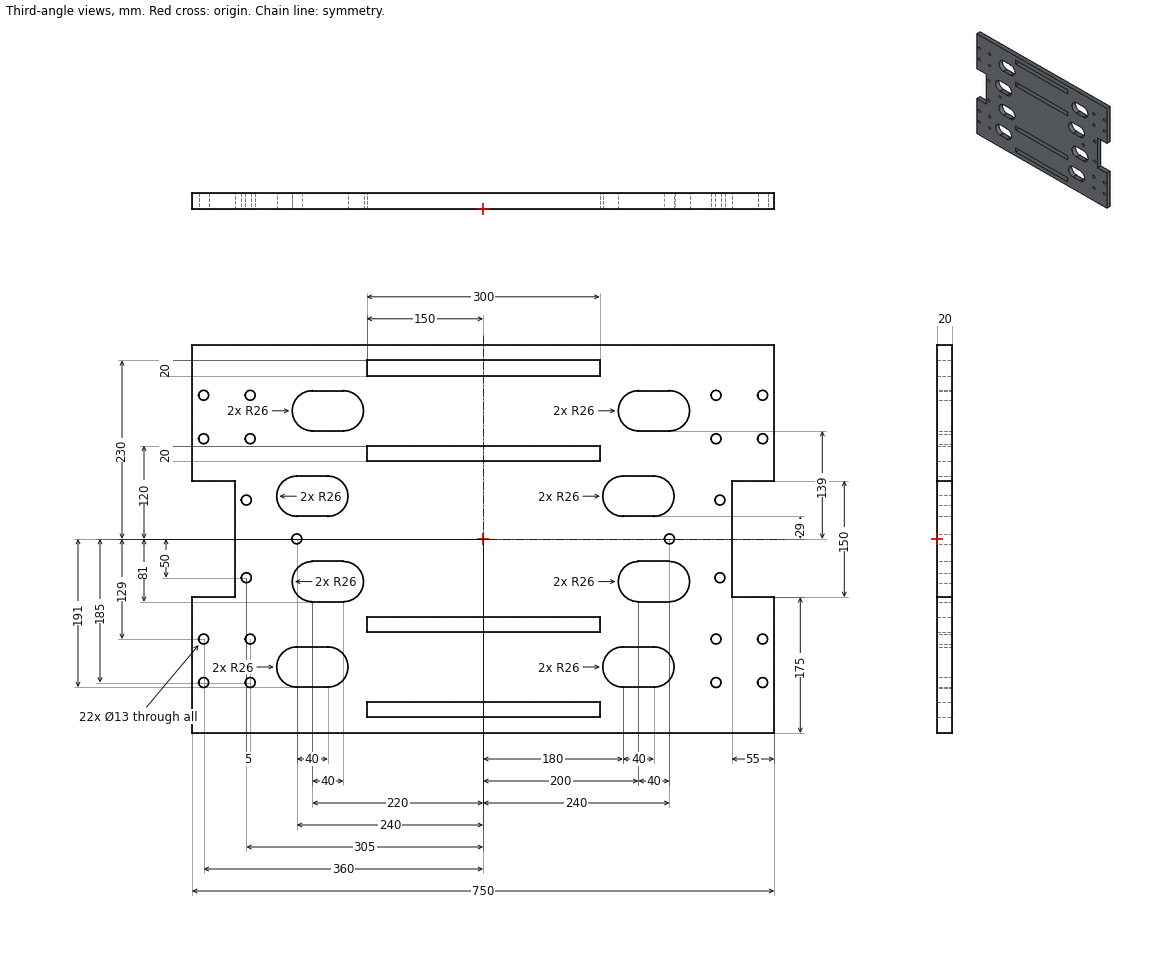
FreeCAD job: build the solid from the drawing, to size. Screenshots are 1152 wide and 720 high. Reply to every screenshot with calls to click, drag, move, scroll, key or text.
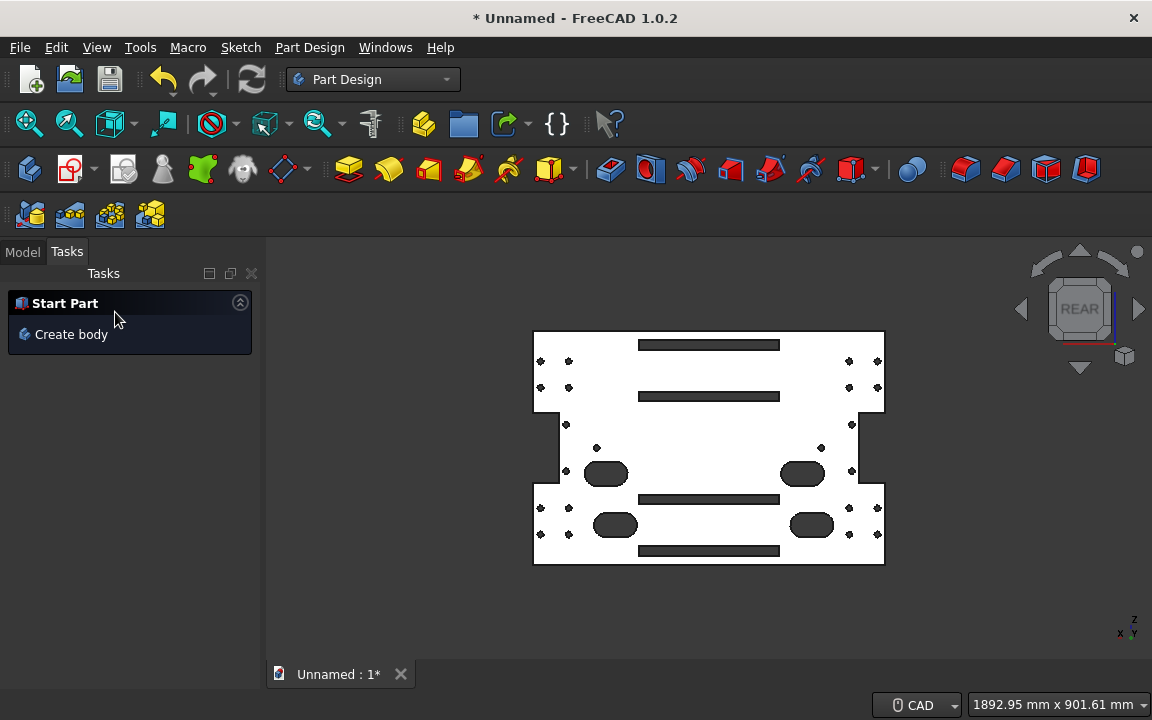
click(709, 447)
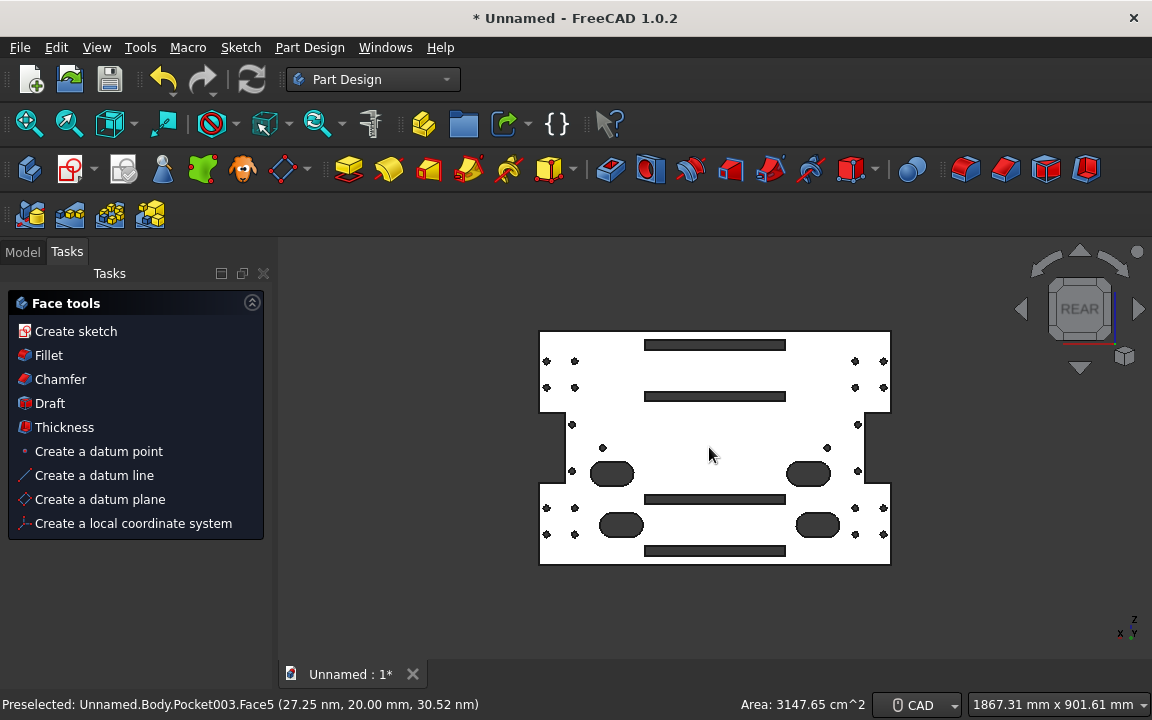
click(70, 170)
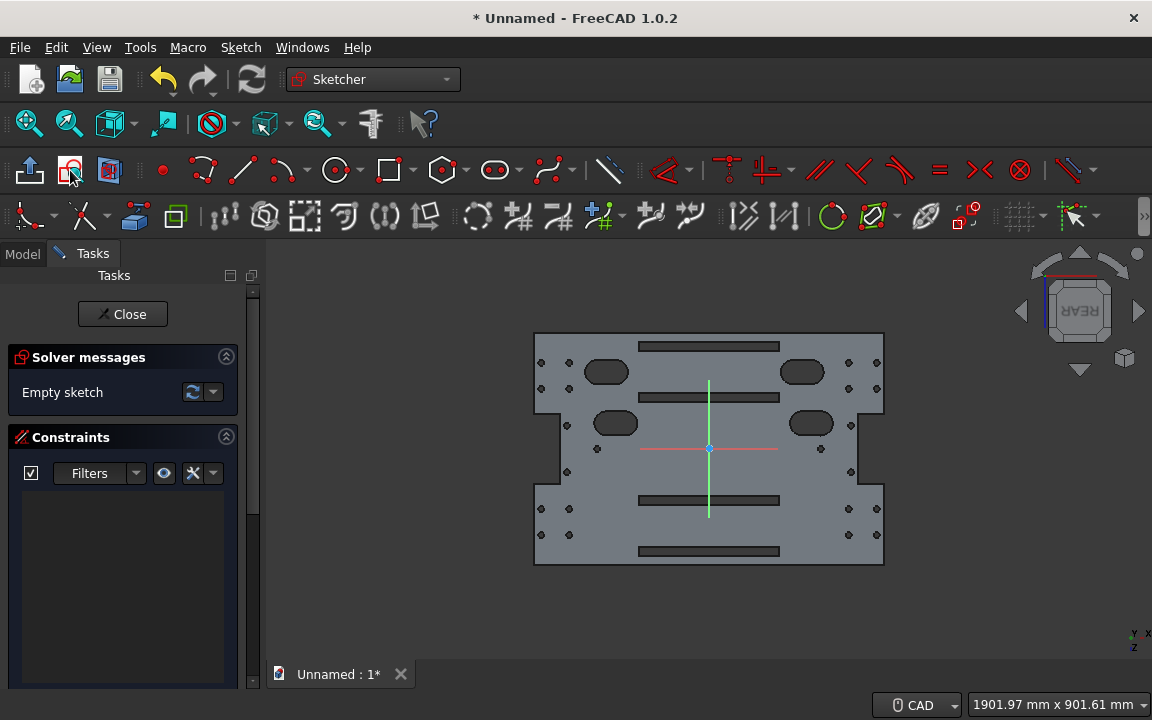
scroll(818, 477, up, 12)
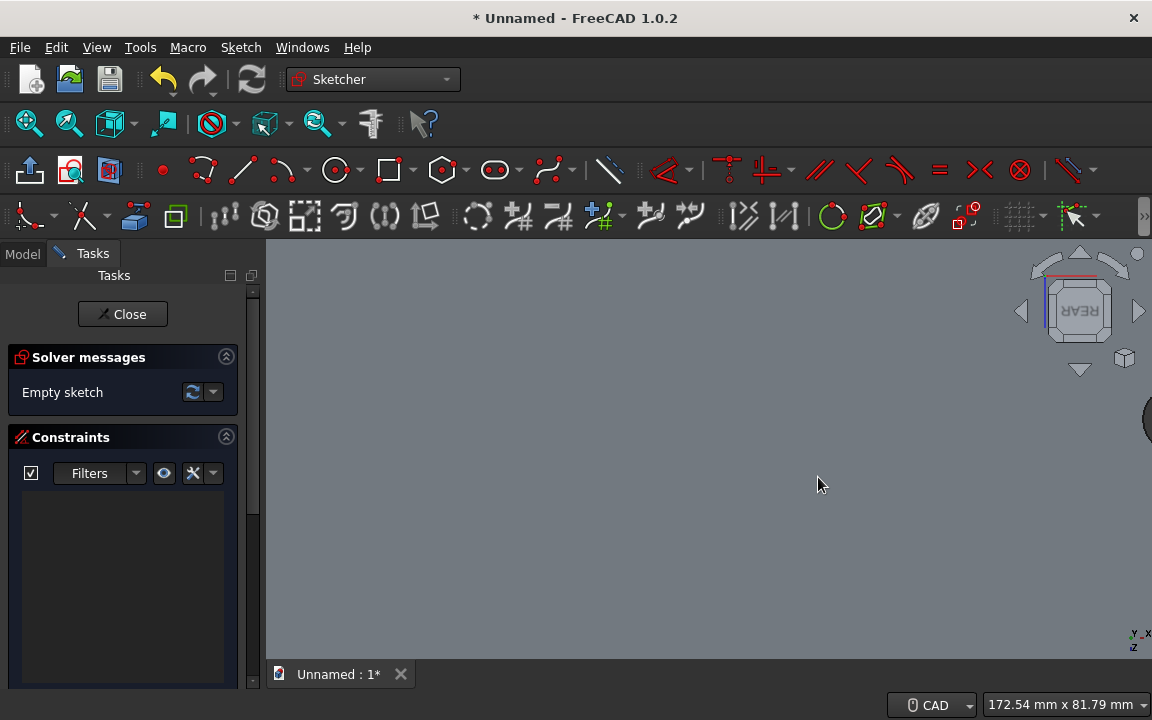
click(496, 170)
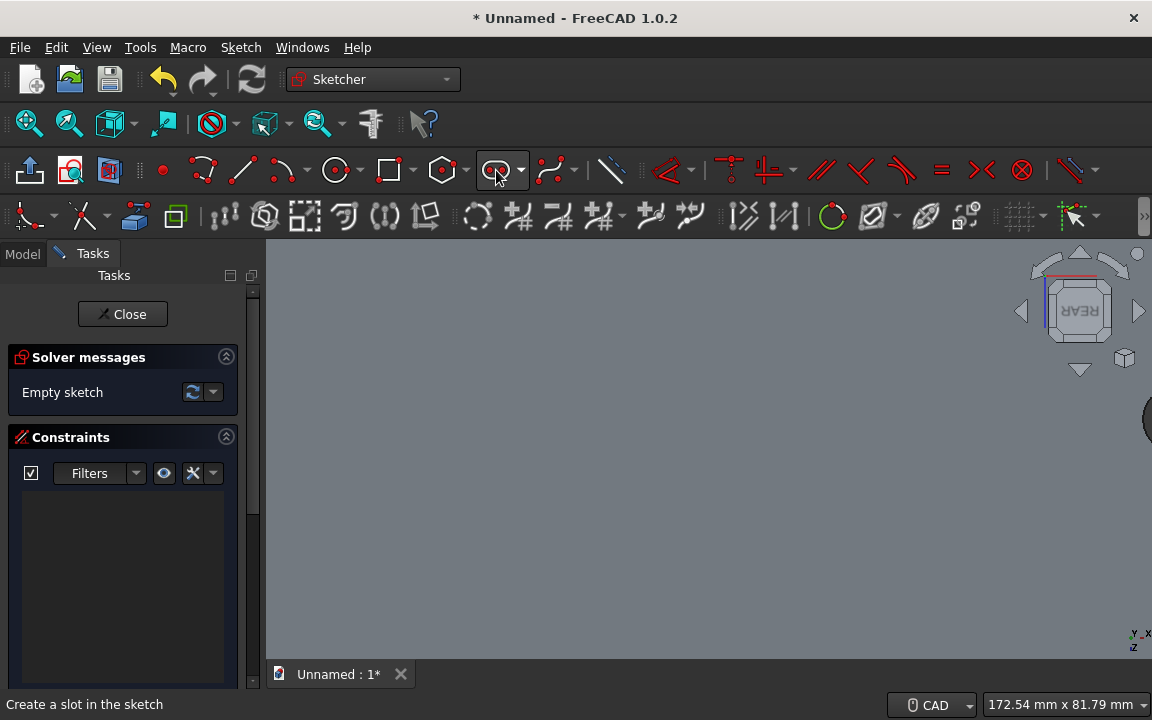
click(535, 445)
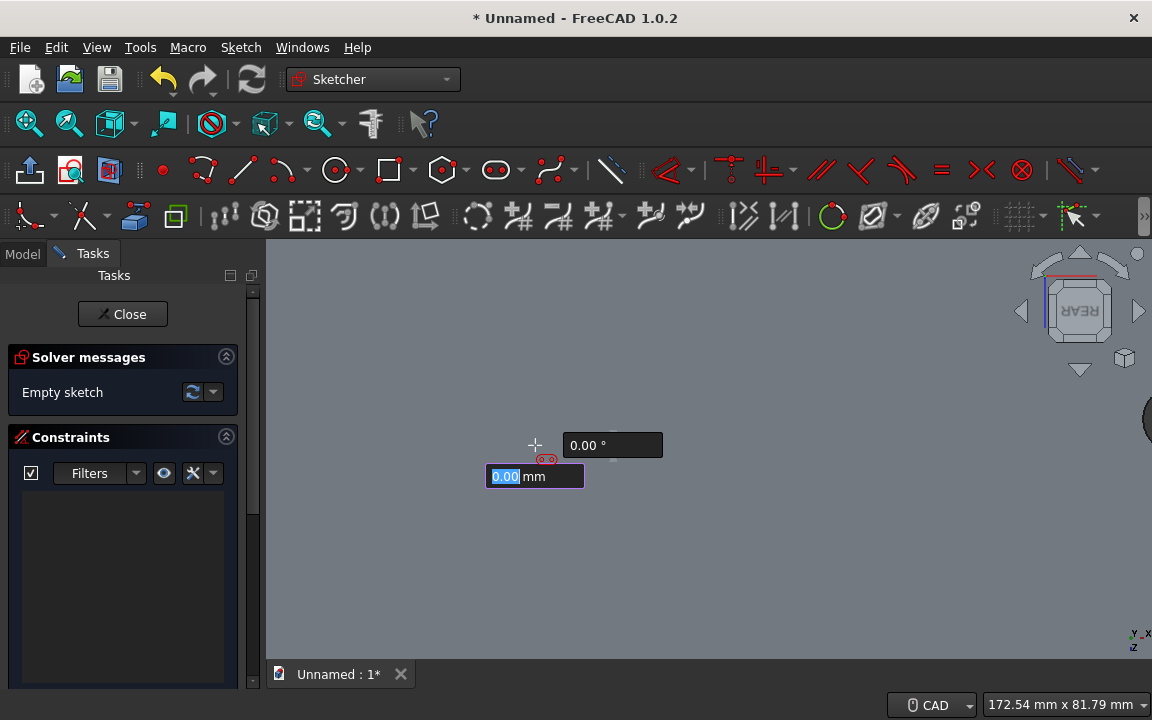
click(740, 445)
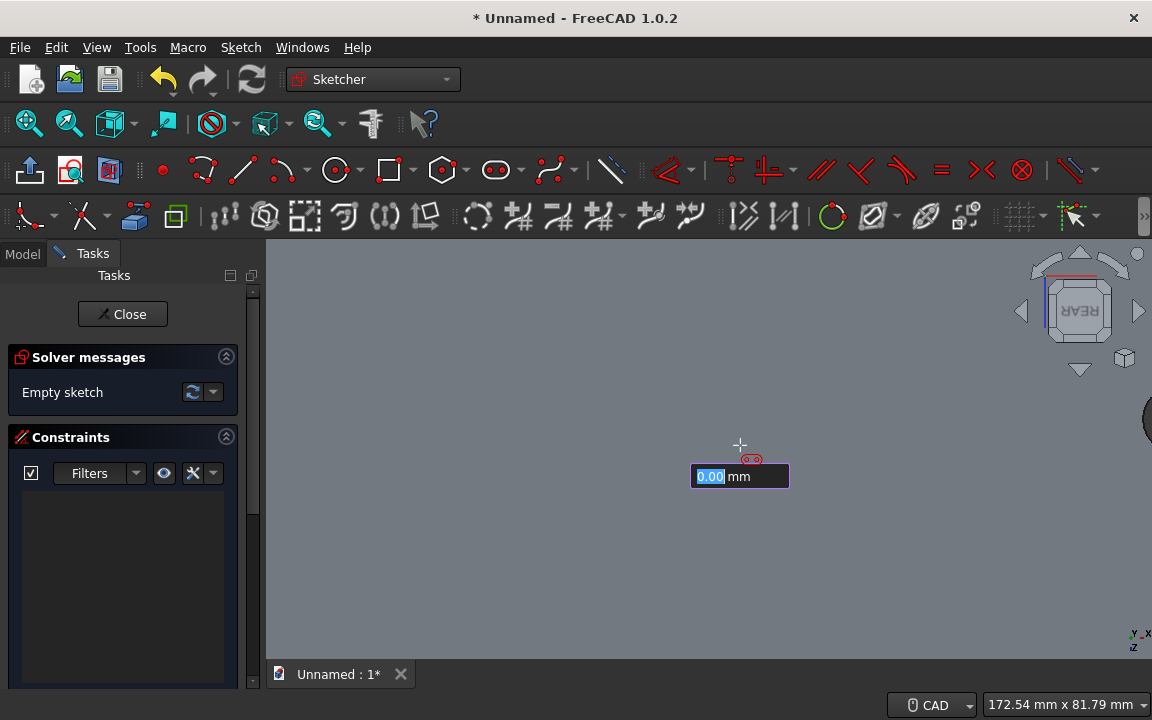
click(637, 312)
key(Escape)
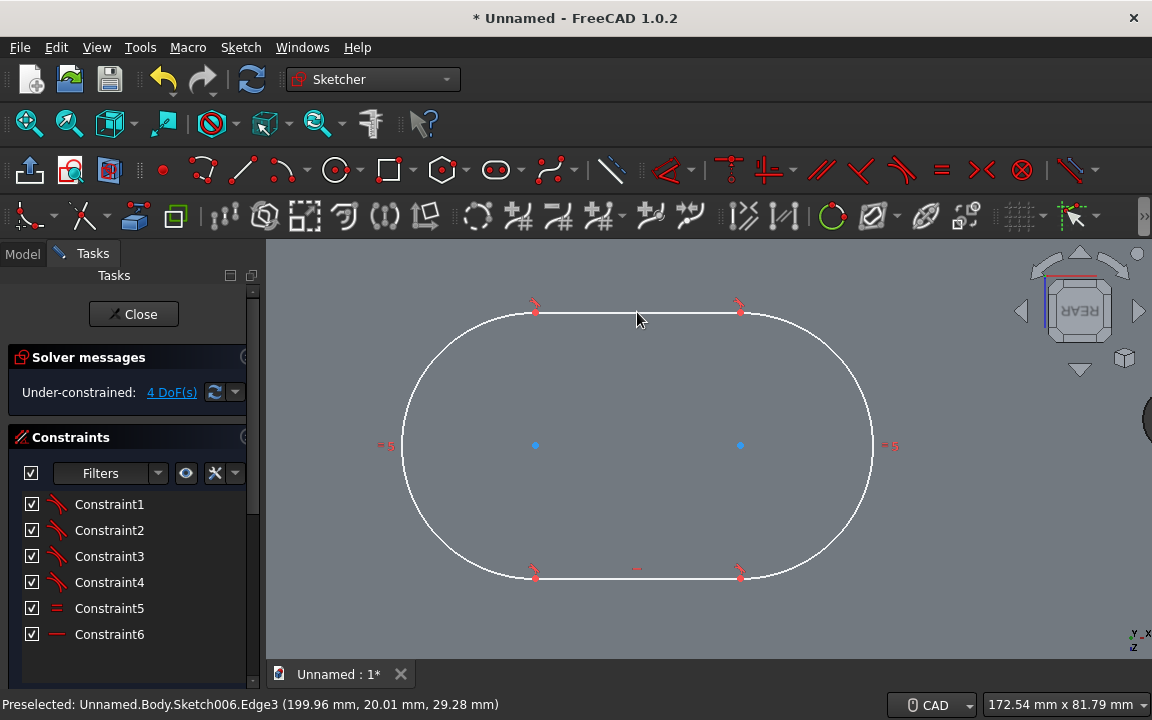
click(666, 170)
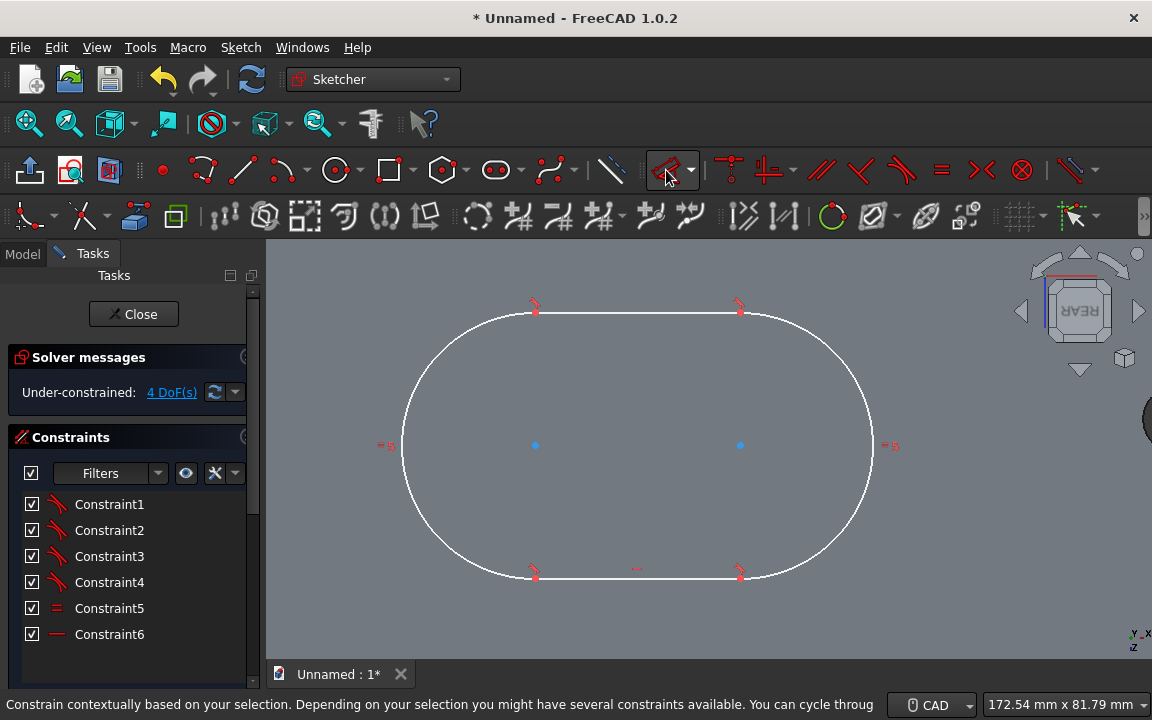
click(427, 368)
click(401, 349)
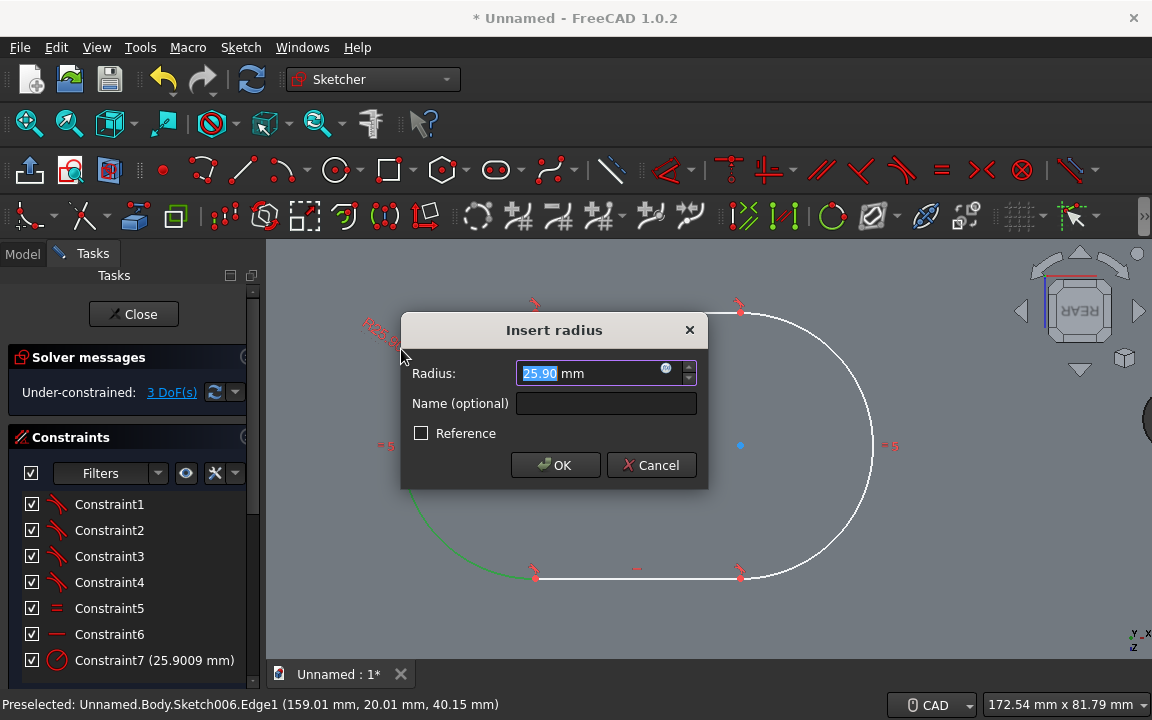
text(26)
key(Return)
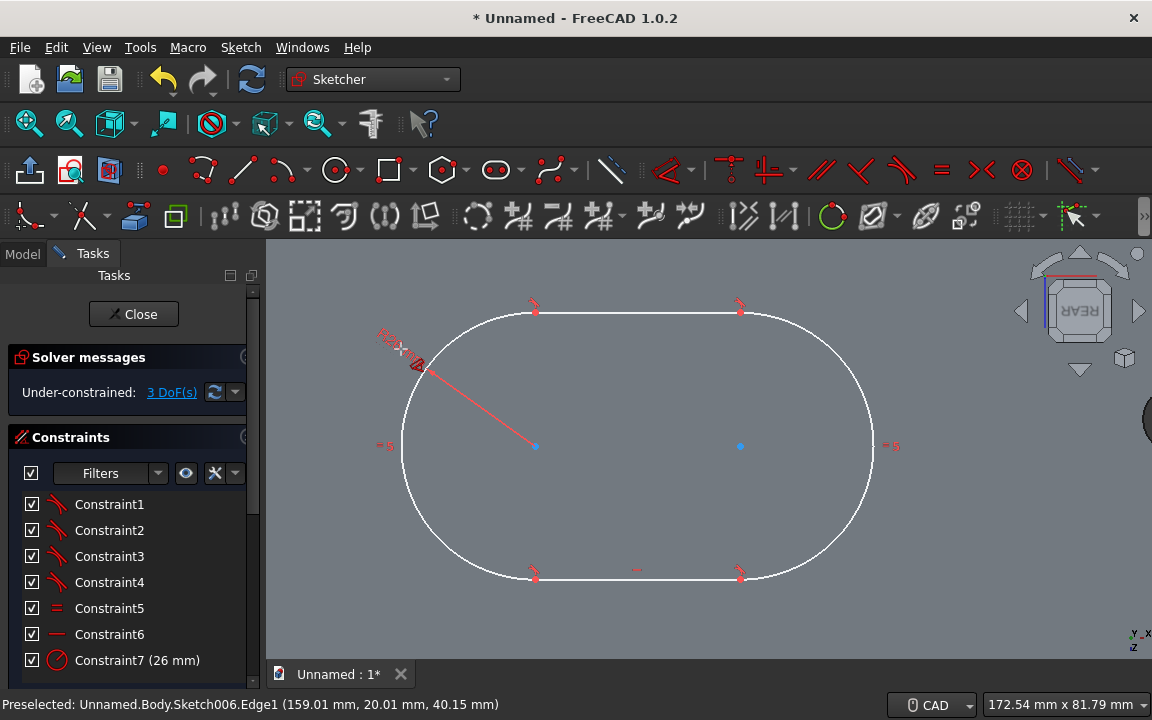
click(596, 313)
click(638, 279)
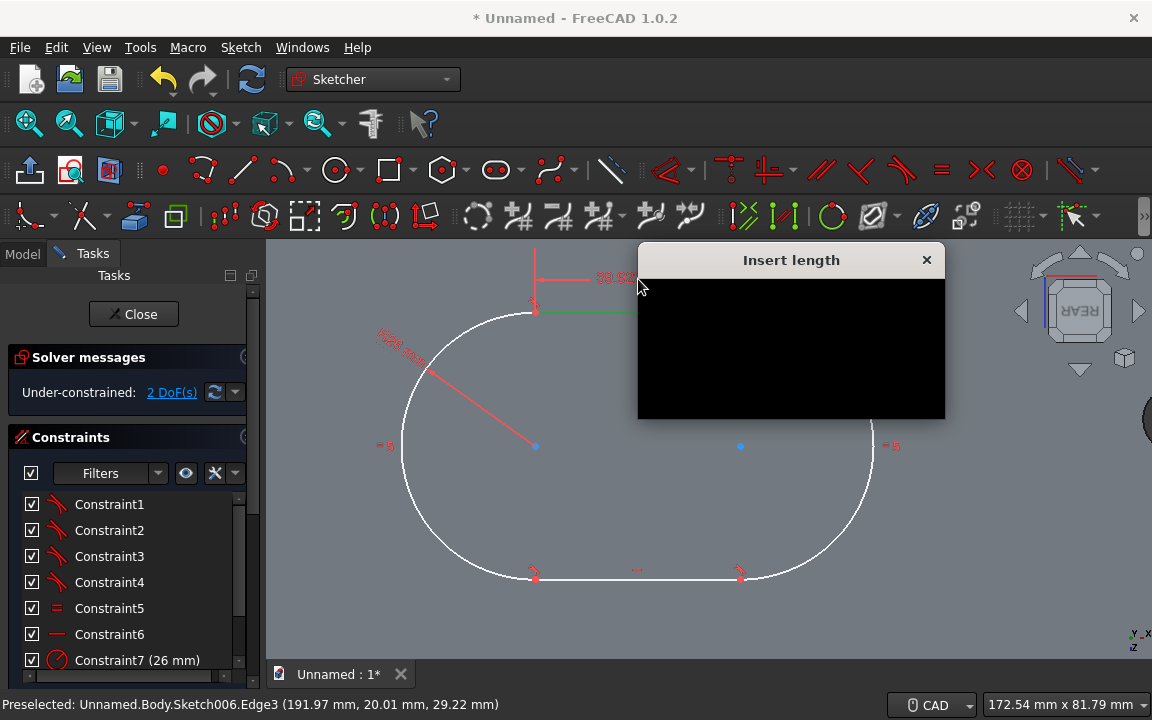
text(40)
key(Return)